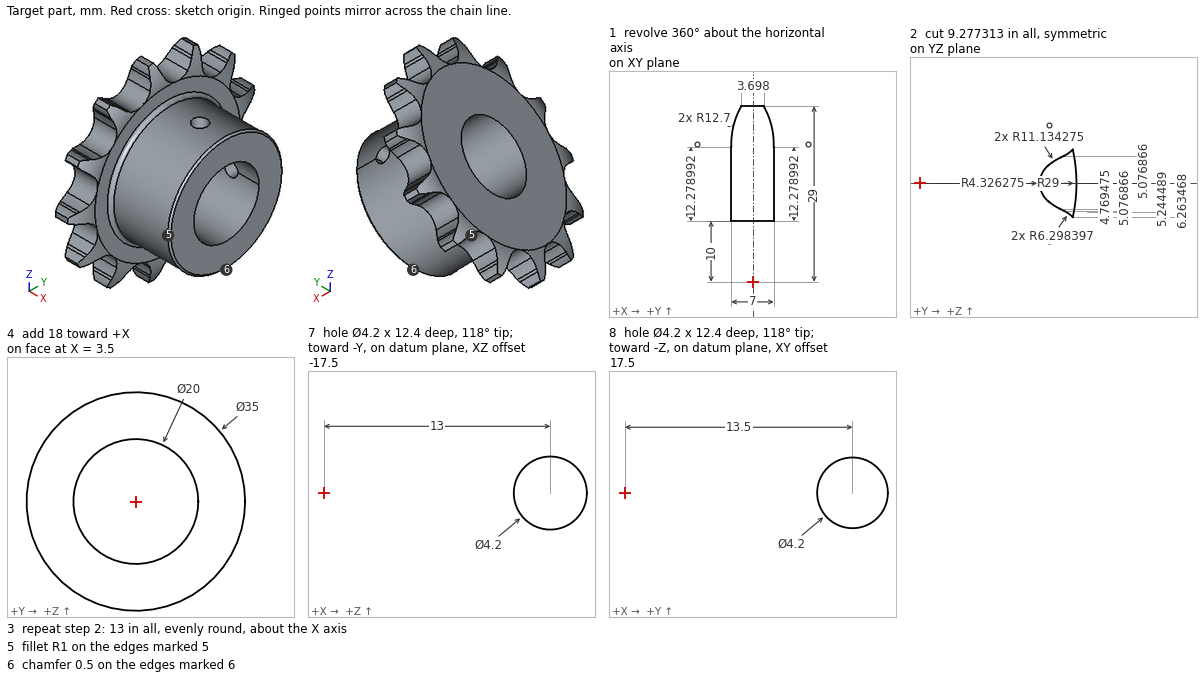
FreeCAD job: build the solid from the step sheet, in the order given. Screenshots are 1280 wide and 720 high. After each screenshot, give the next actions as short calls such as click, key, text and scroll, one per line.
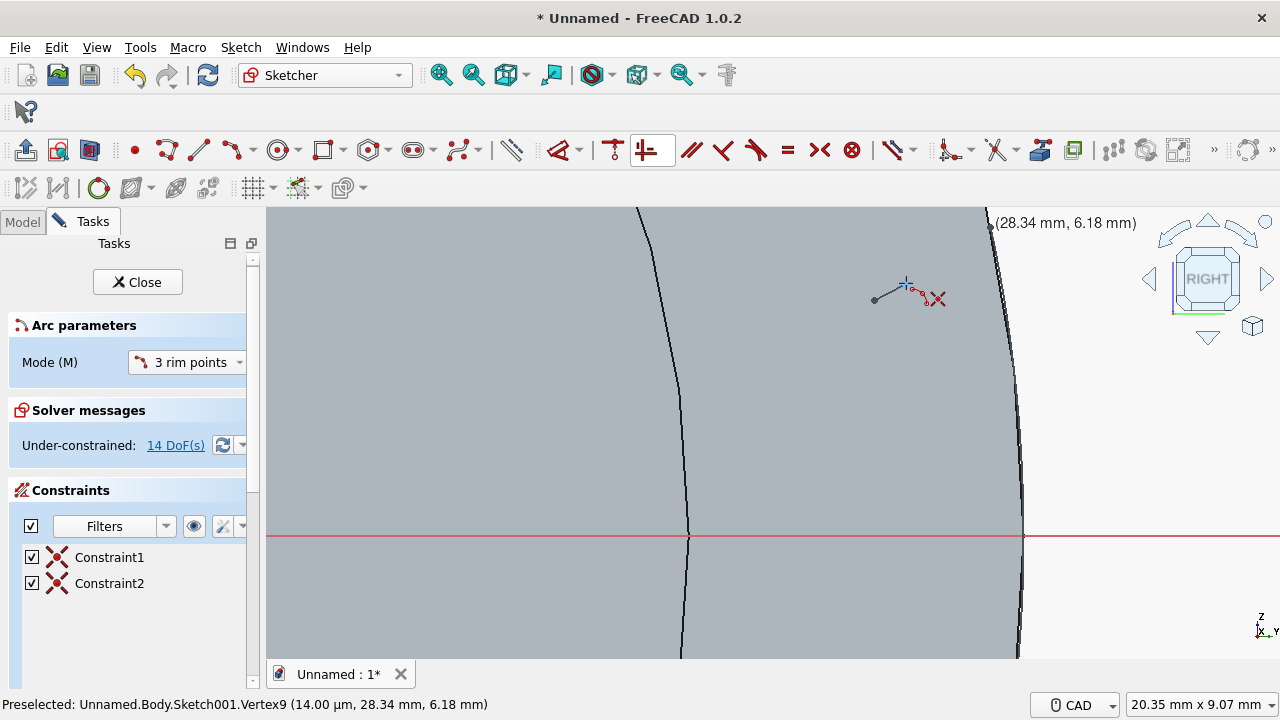
click(905, 284)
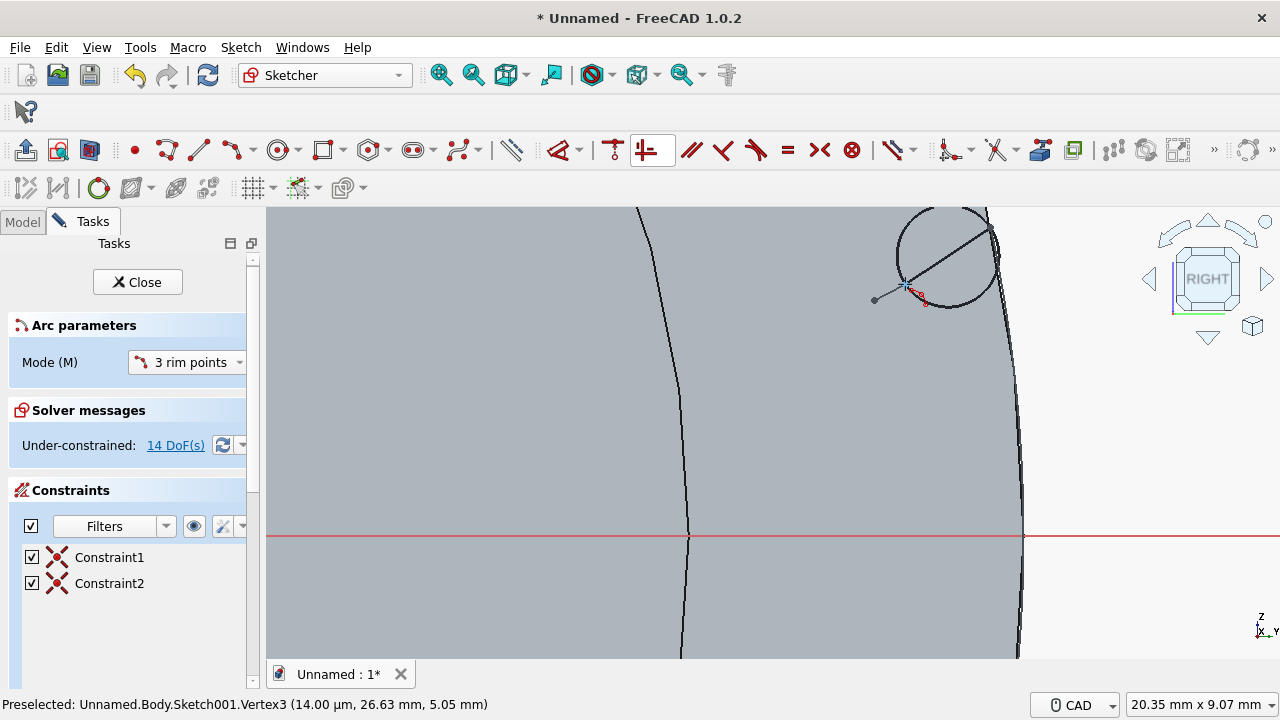
scroll(950, 257, up, 7)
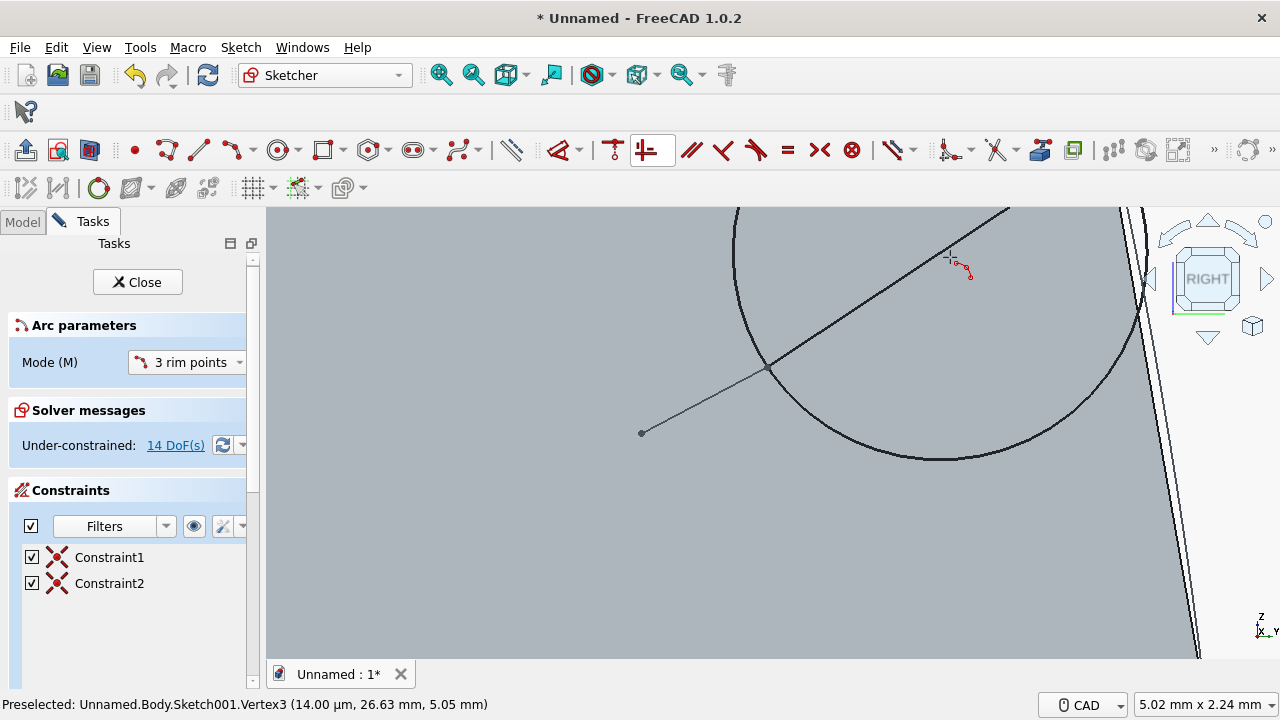
click(949, 256)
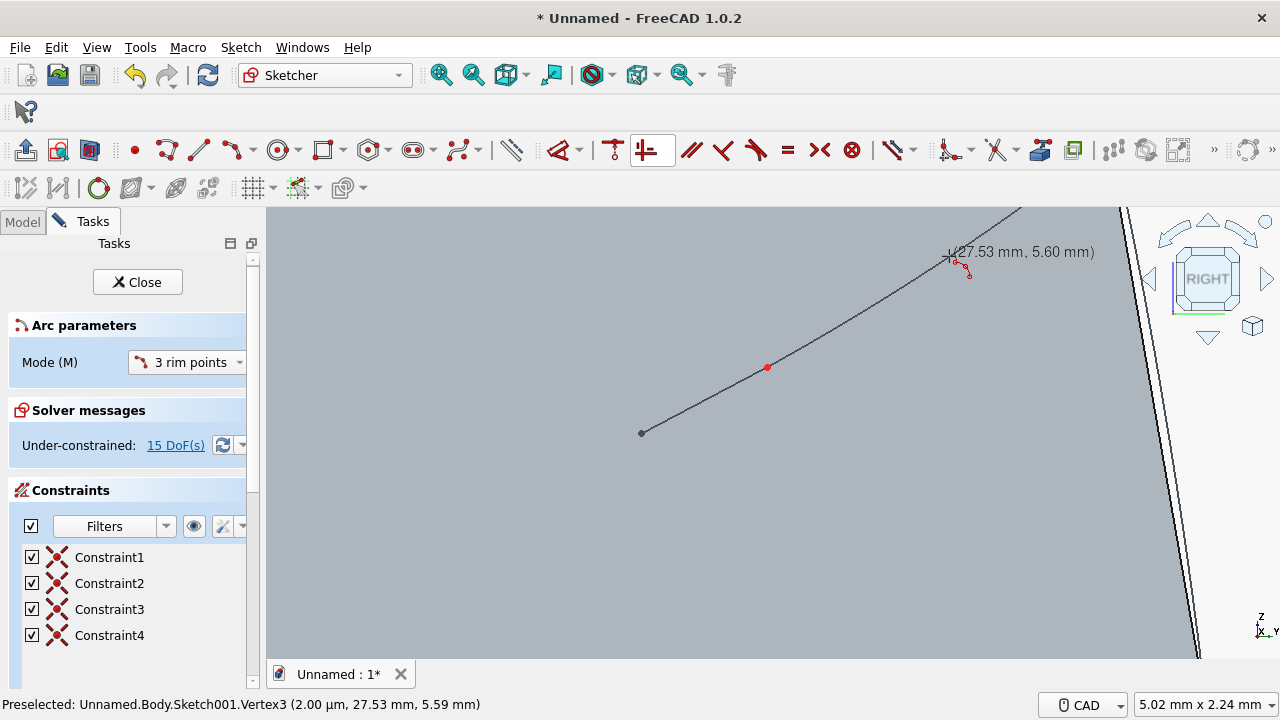
scroll(943, 338, down, 12)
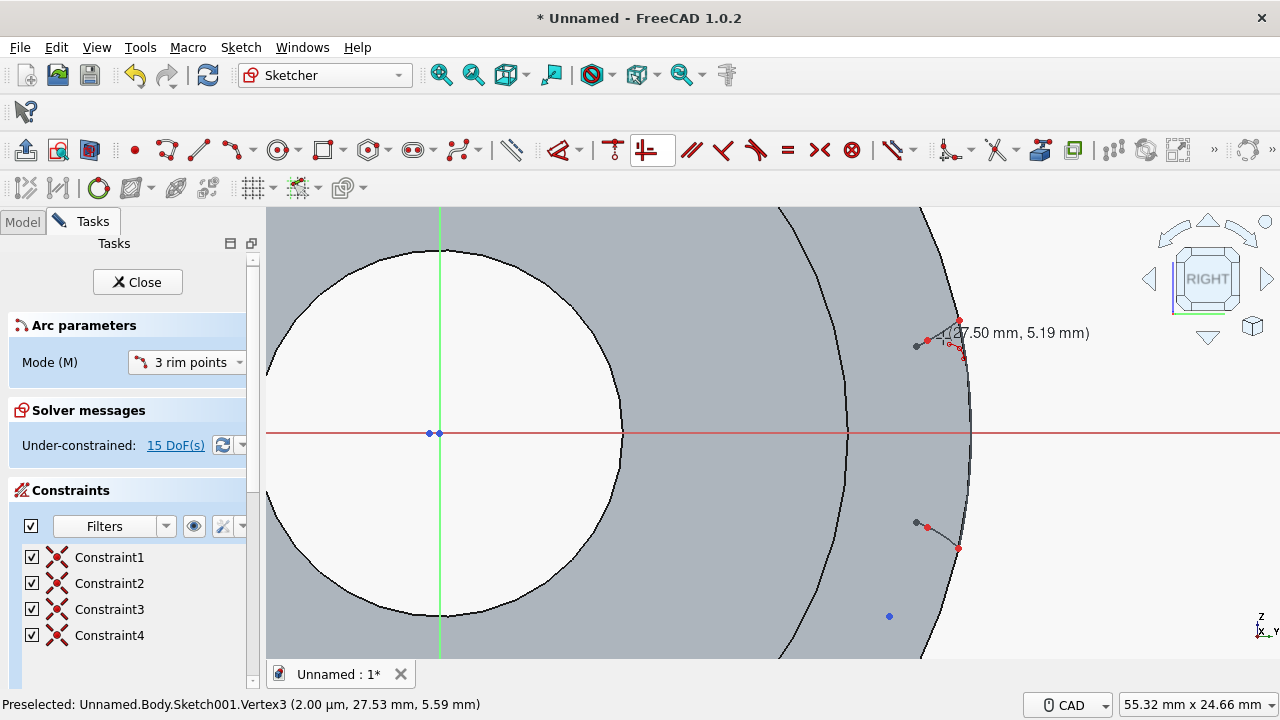
scroll(916, 346, up, 5)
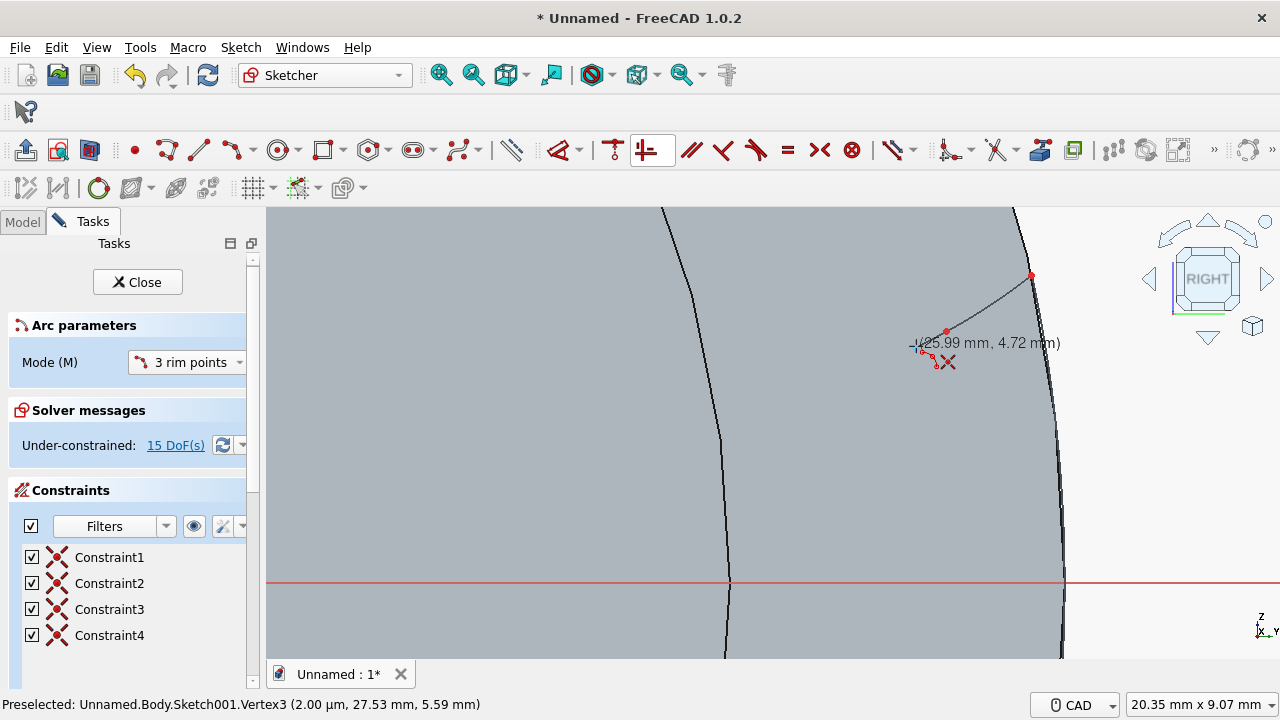
click(916, 348)
click(804, 417)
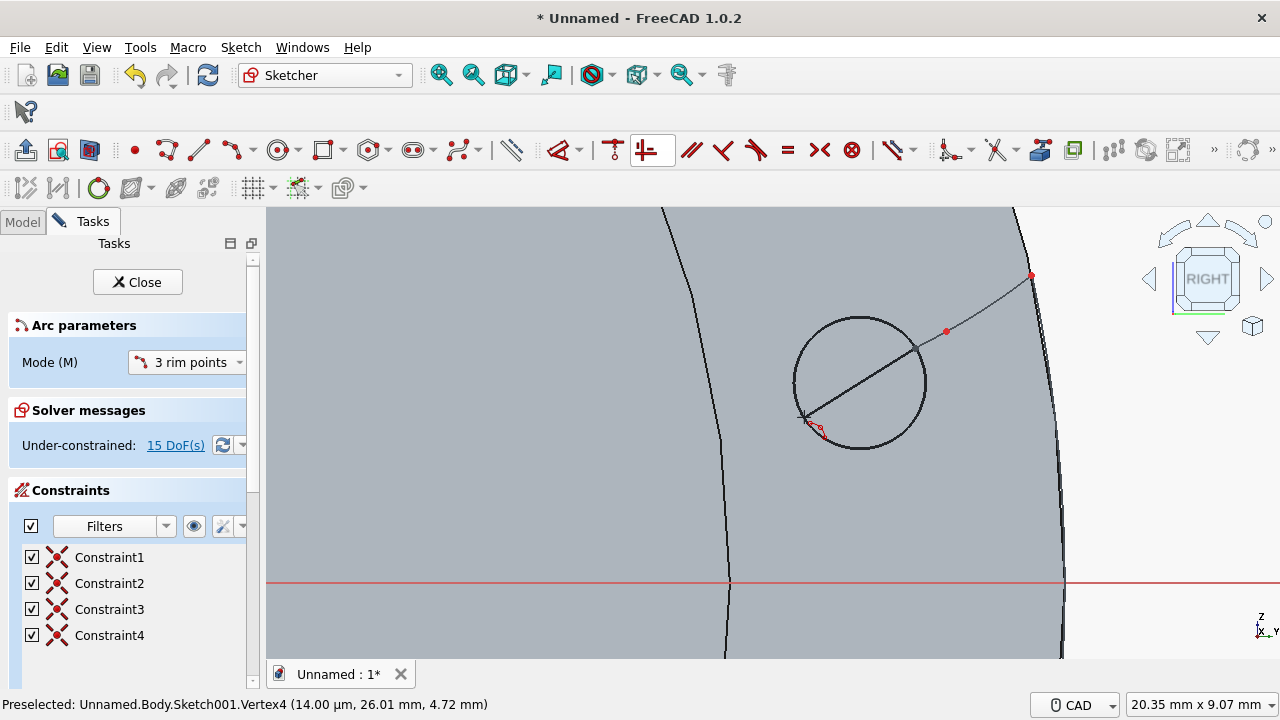
scroll(858, 378, up, 7)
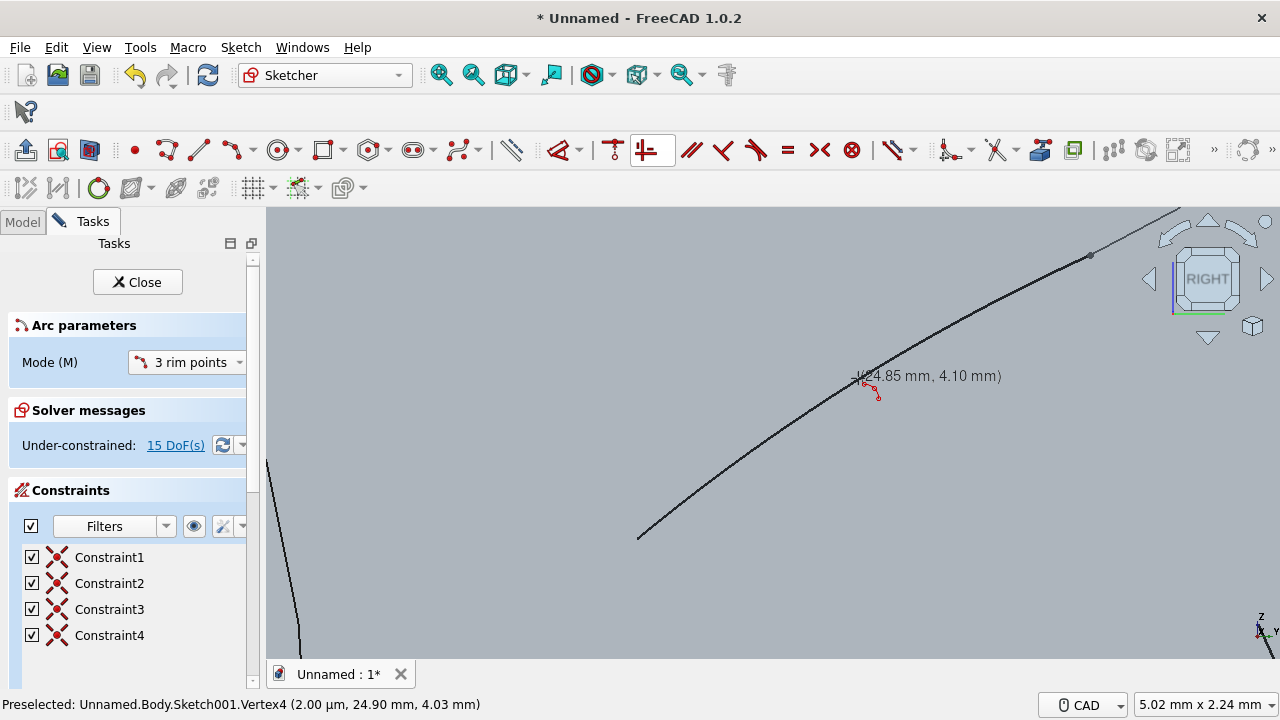
click(856, 377)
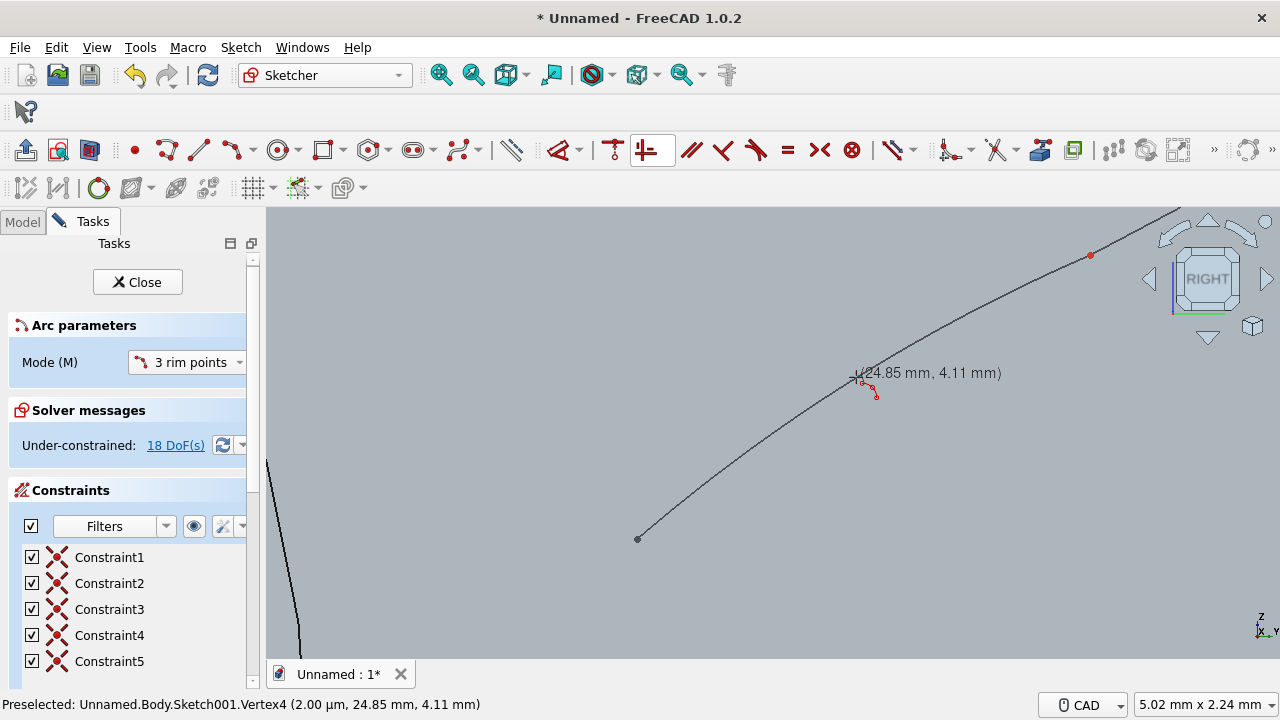
scroll(898, 356, down, 12)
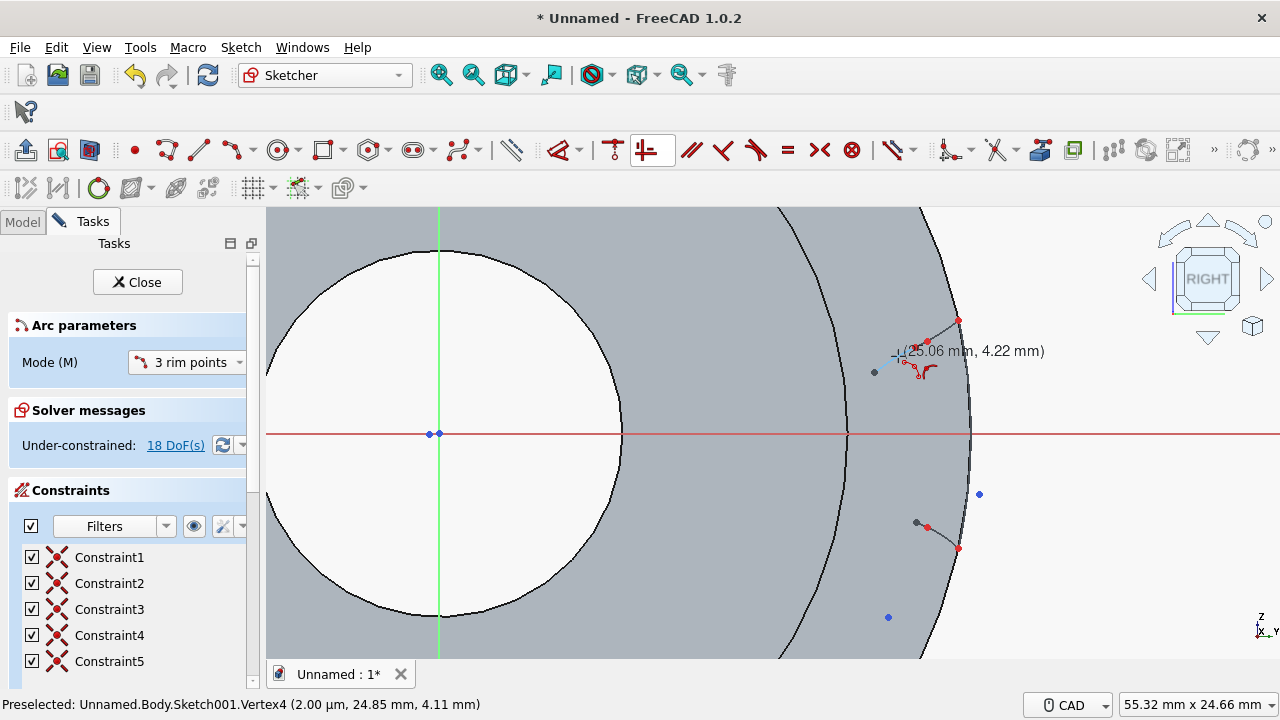
click(875, 373)
click(875, 495)
click(851, 406)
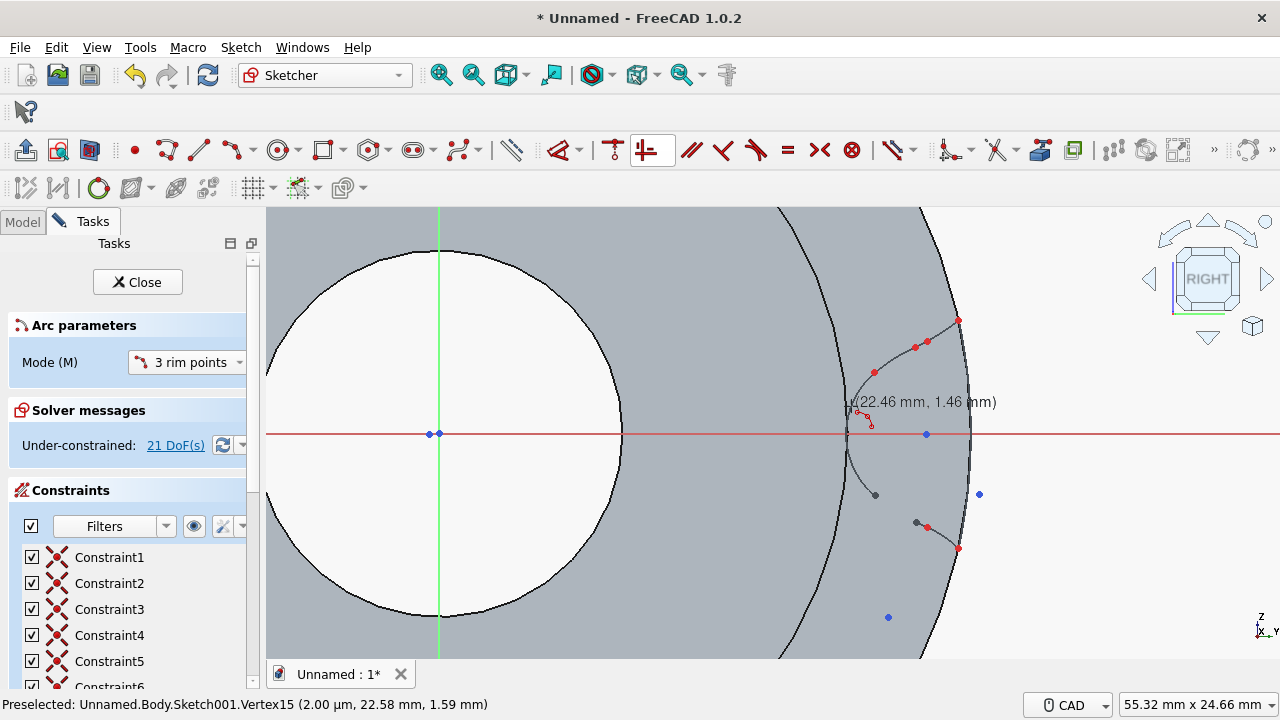
click(875, 496)